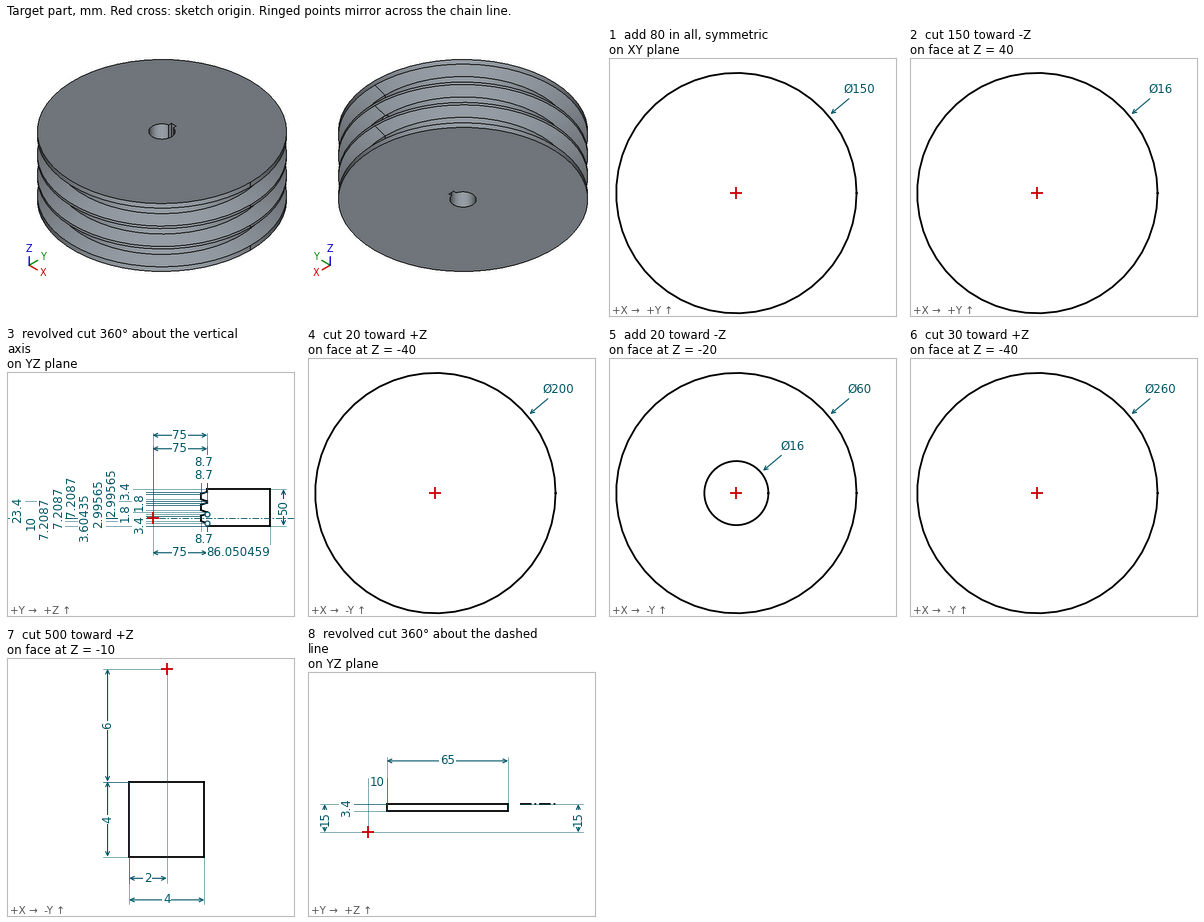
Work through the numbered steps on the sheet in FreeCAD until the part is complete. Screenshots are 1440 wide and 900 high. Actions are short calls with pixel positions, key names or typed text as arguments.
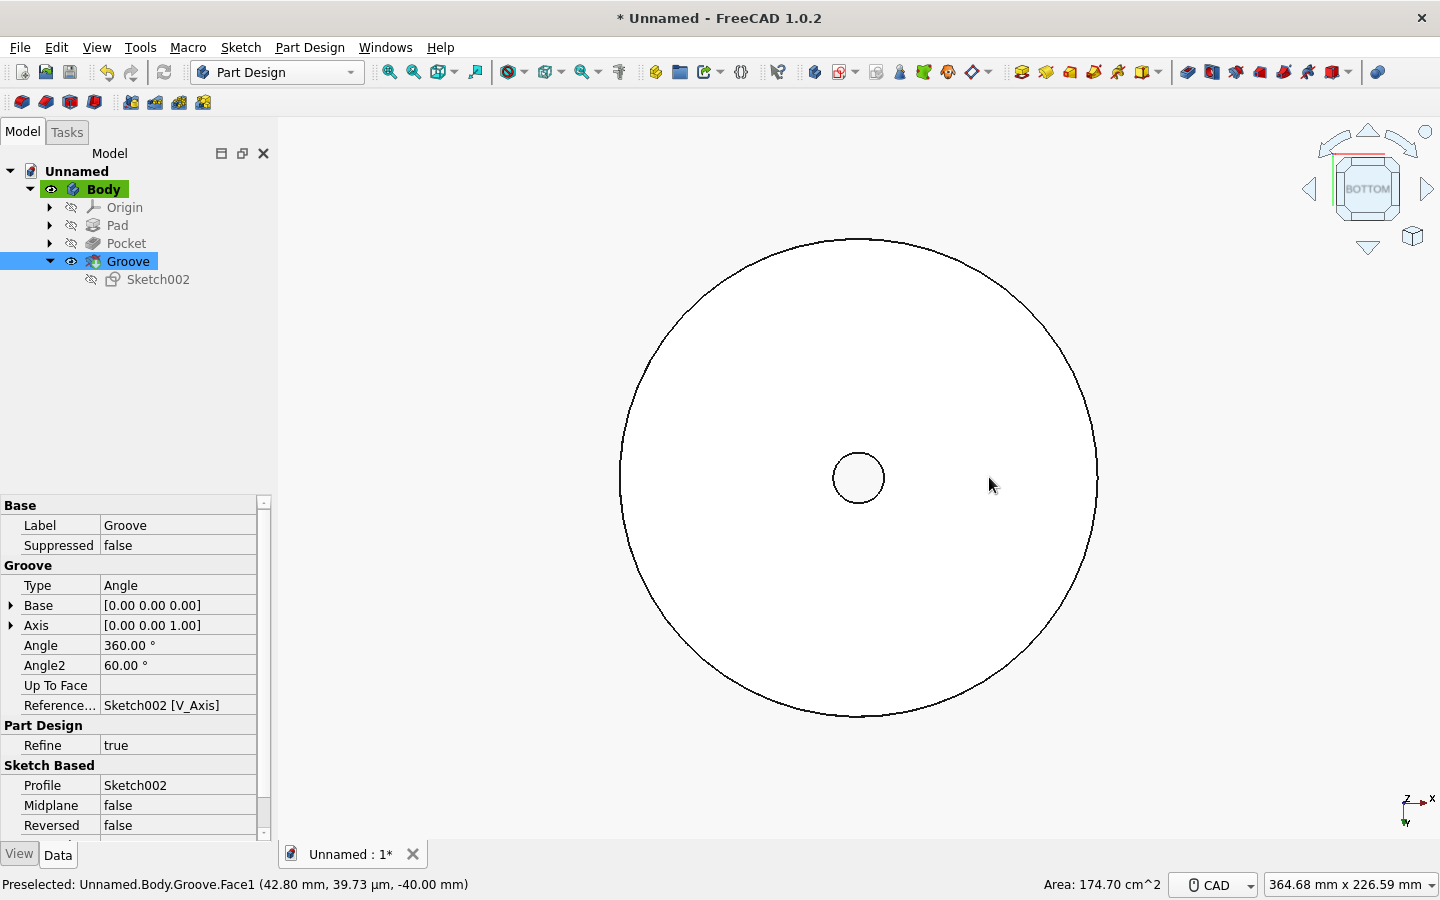
click(840, 72)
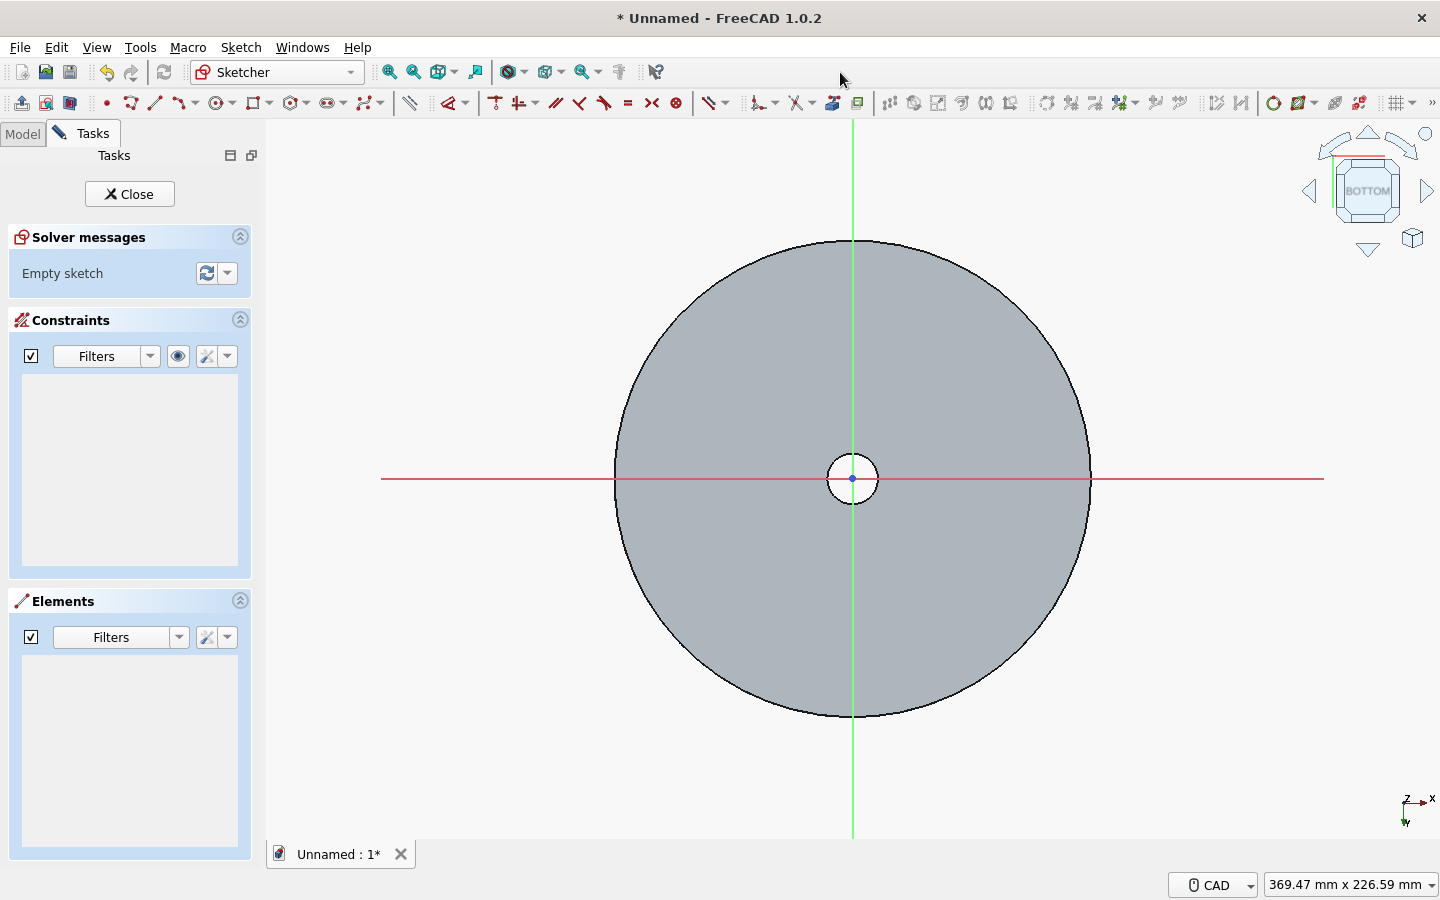
scroll(646, 479, down, 2)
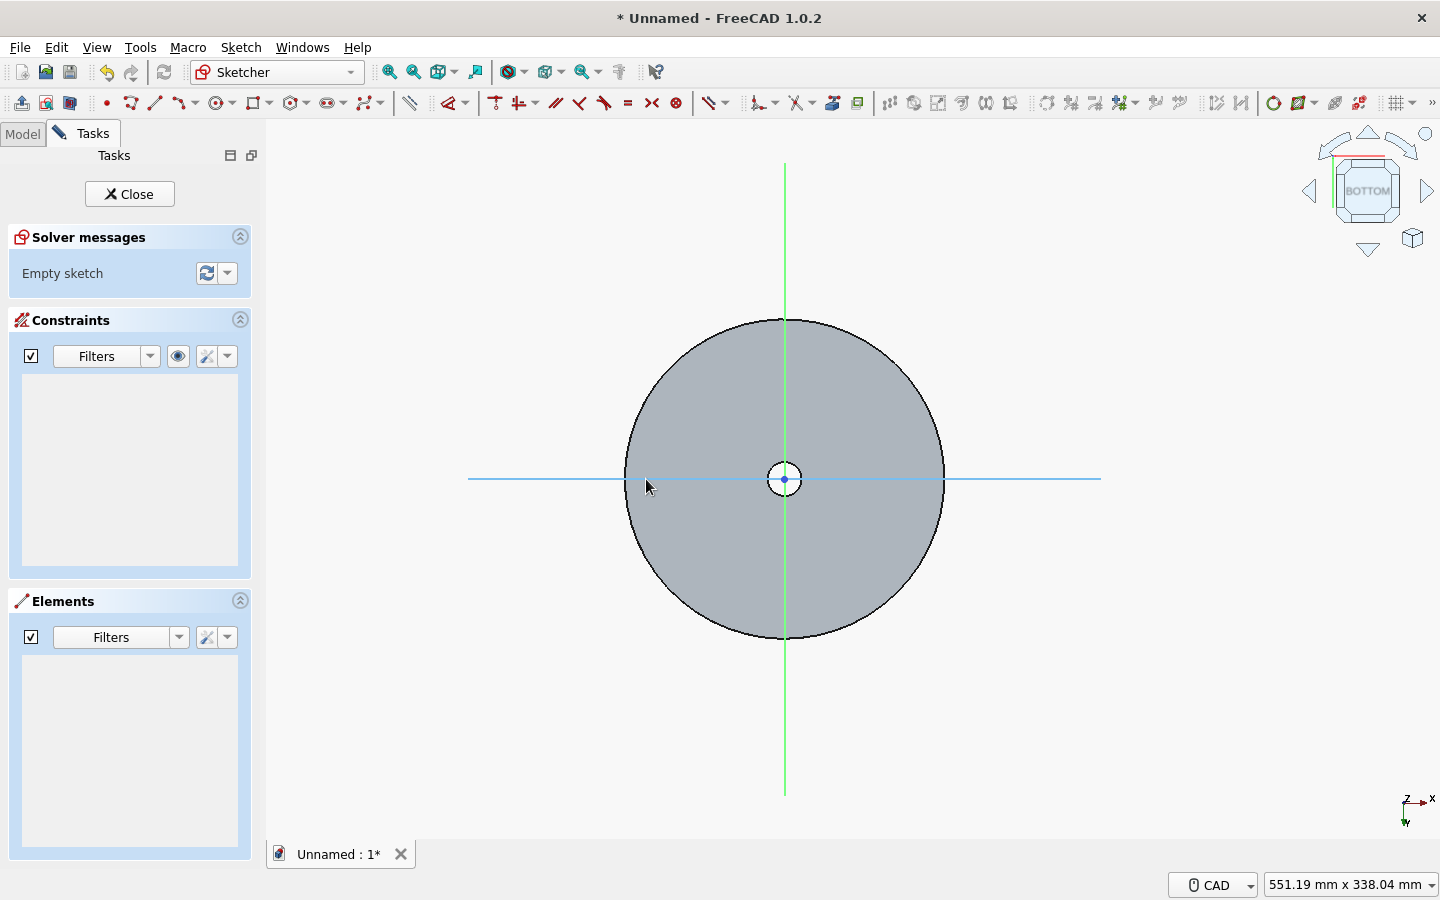
key(g)
key(c)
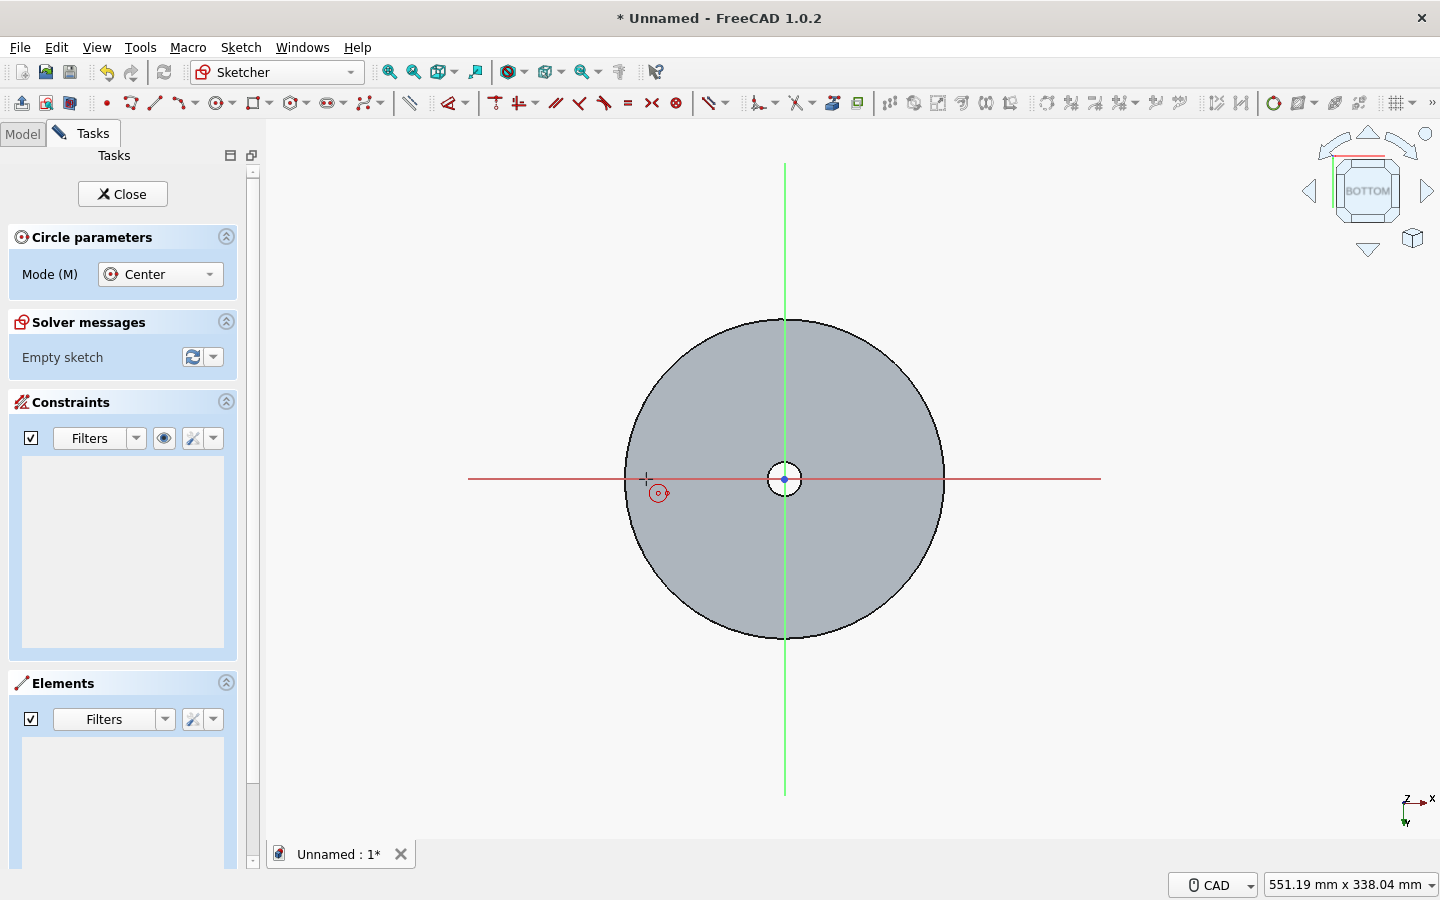
click(785, 479)
click(935, 328)
key(Escape)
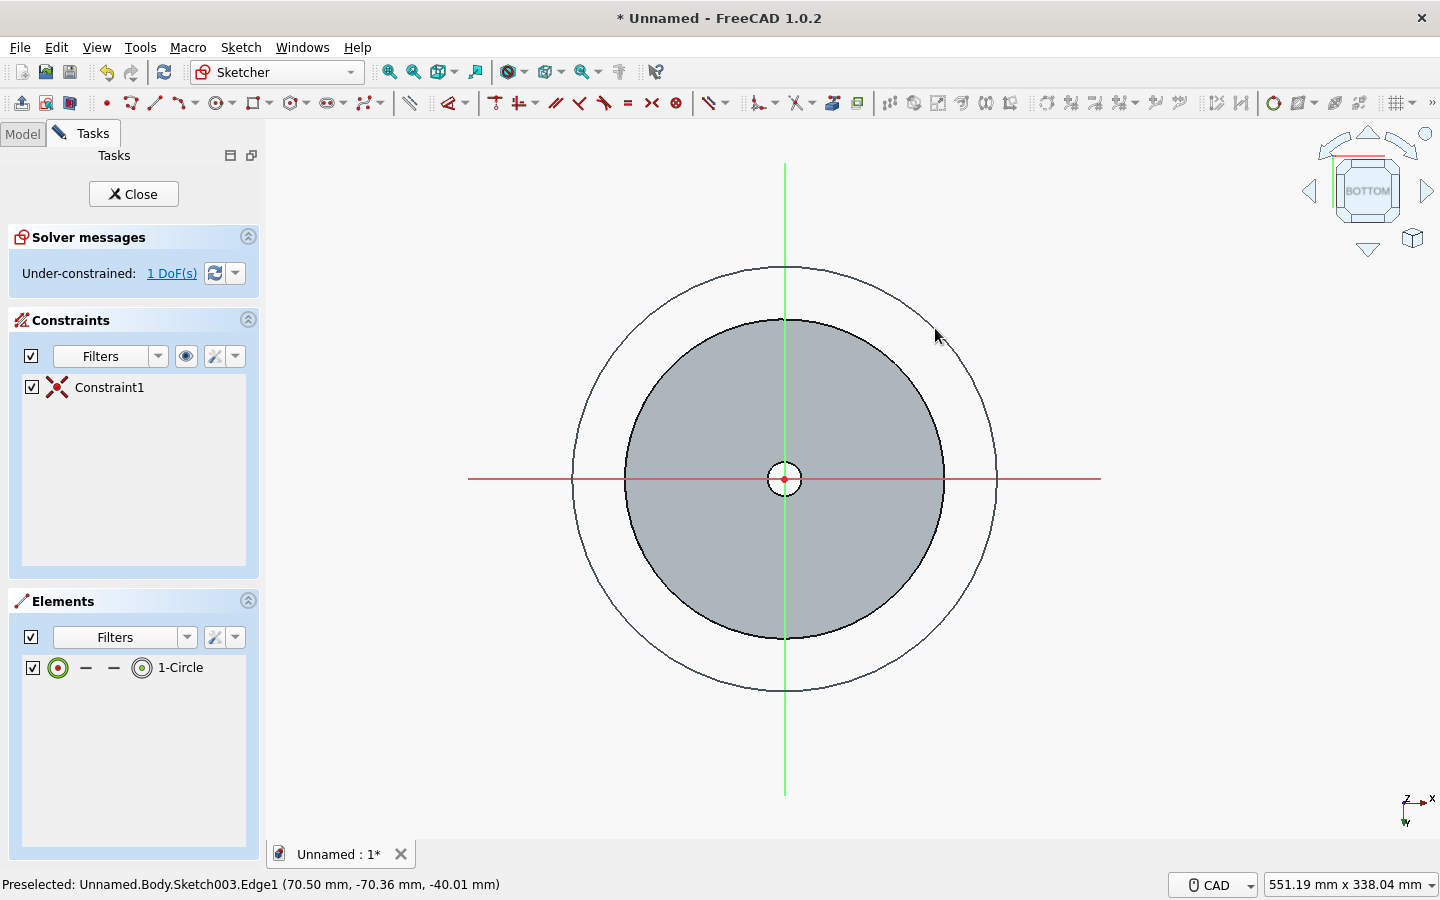
key(d)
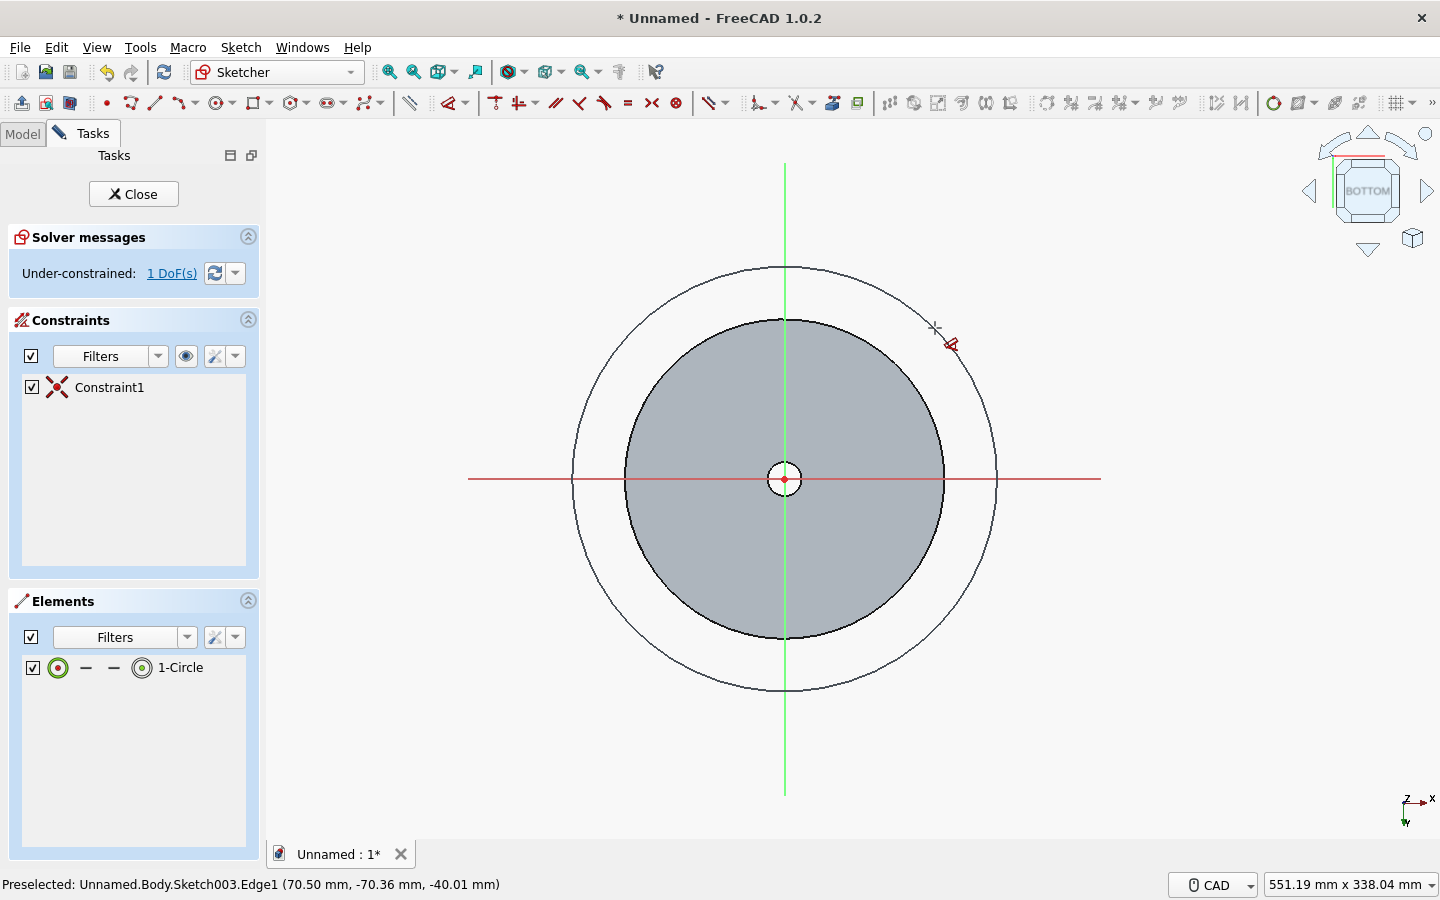
click(934, 328)
click(956, 305)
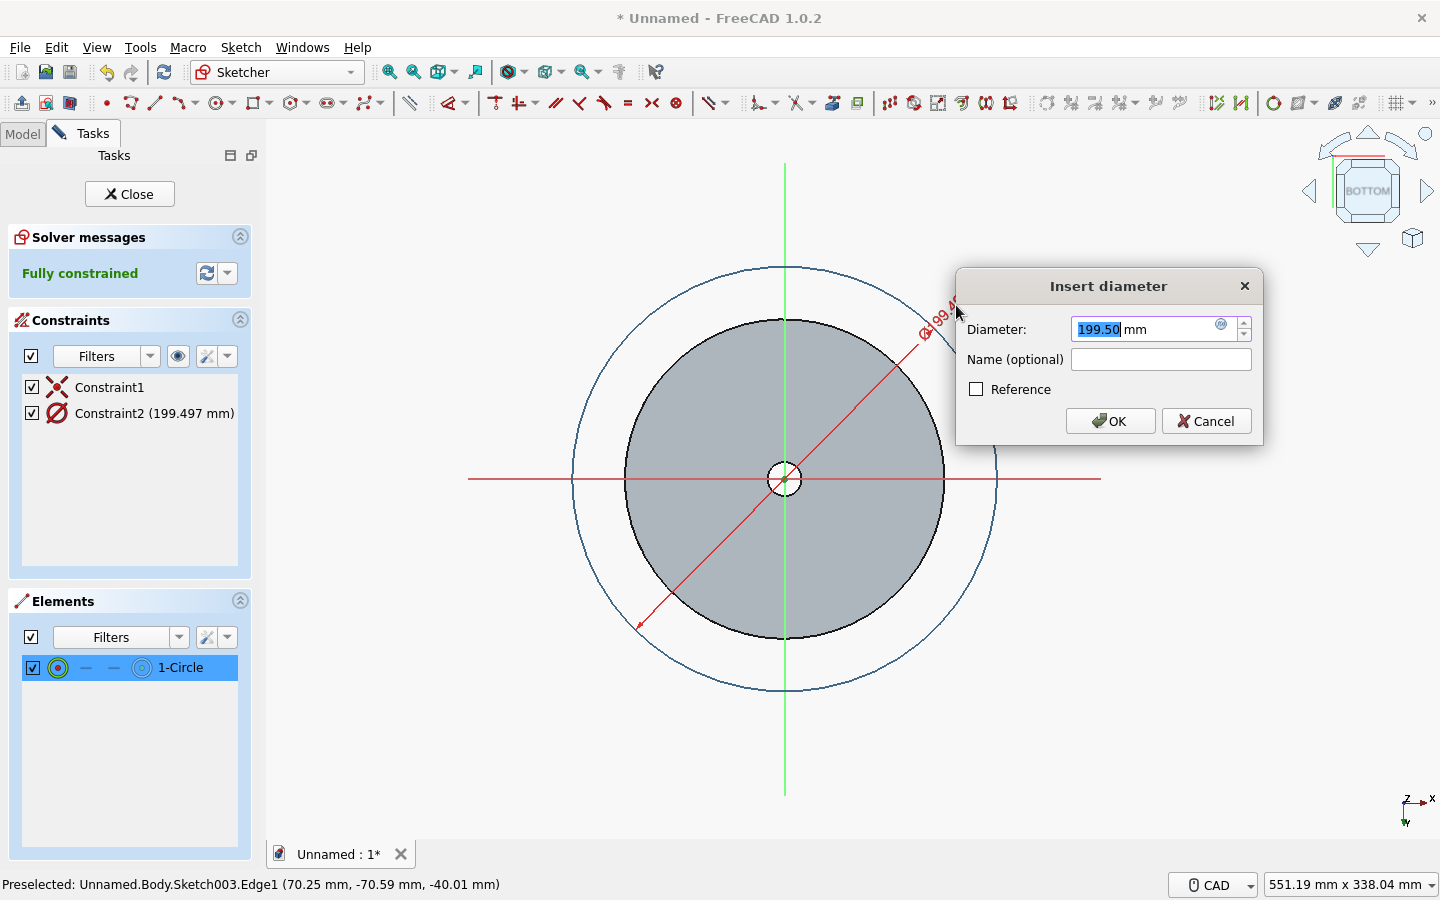
text(200)
key(Return)
key(Escape)